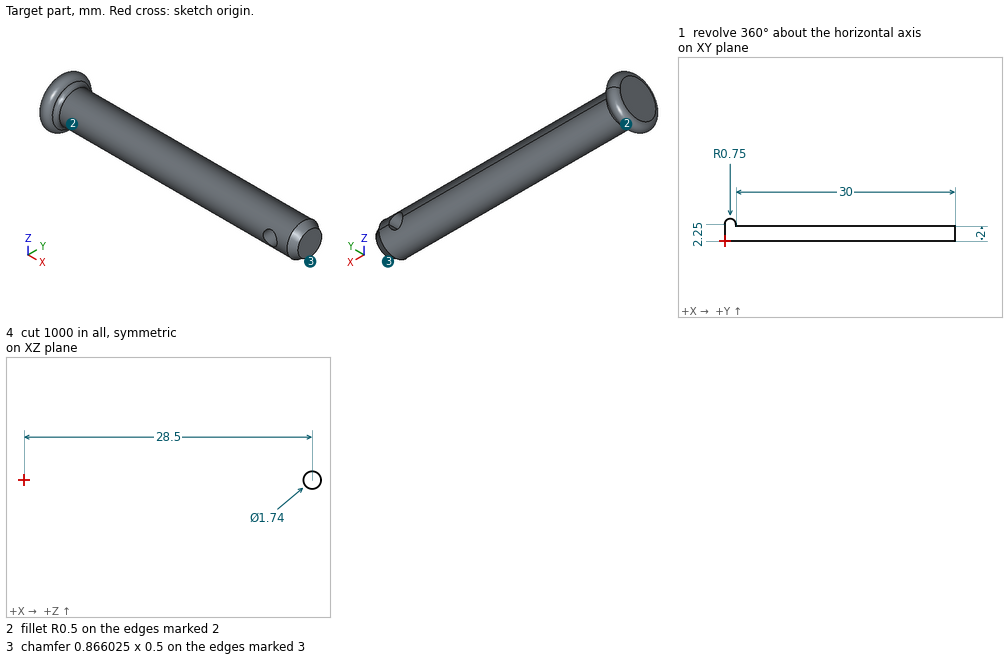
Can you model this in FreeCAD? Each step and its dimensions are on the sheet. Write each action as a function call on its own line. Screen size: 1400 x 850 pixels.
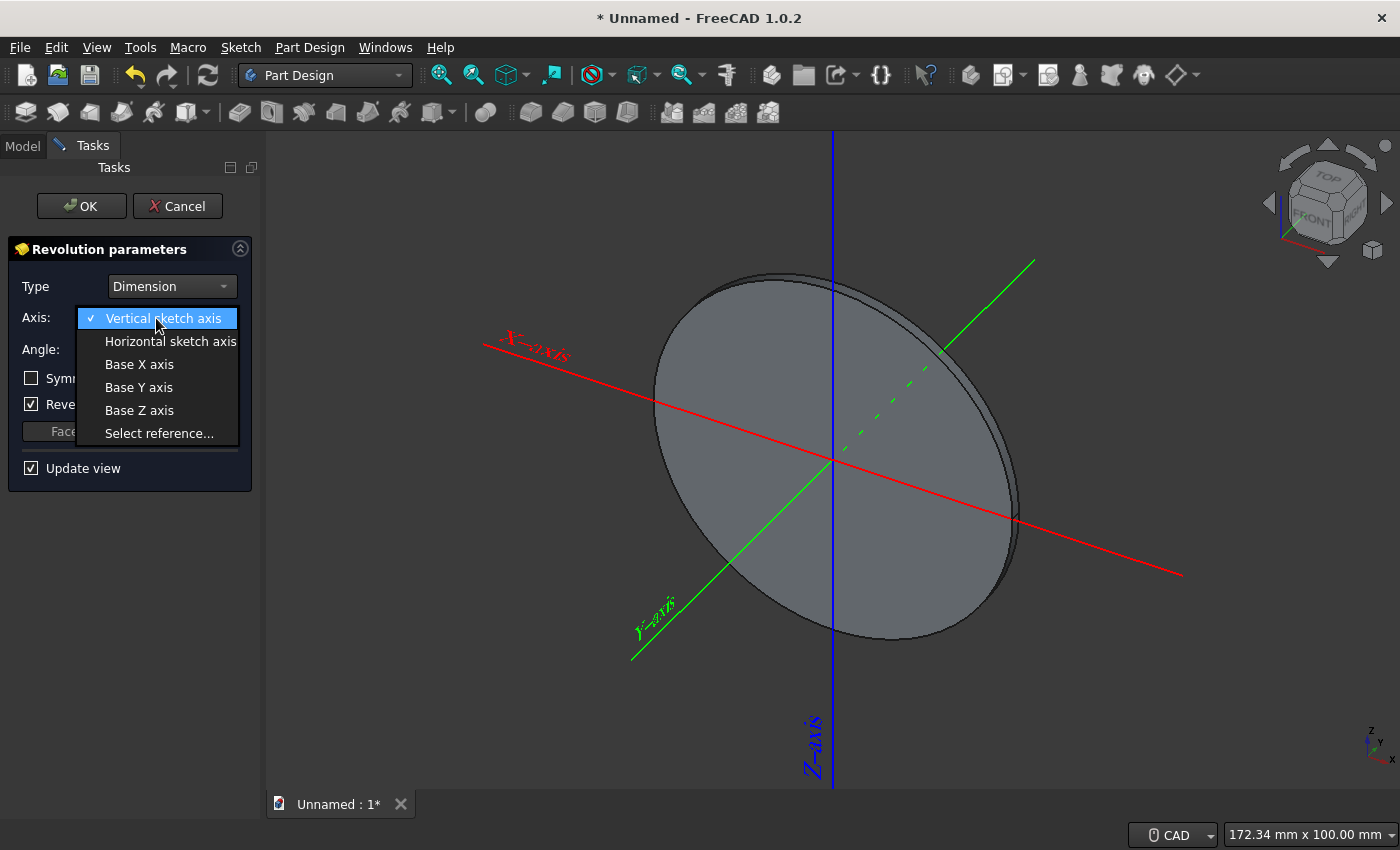
click(156, 342)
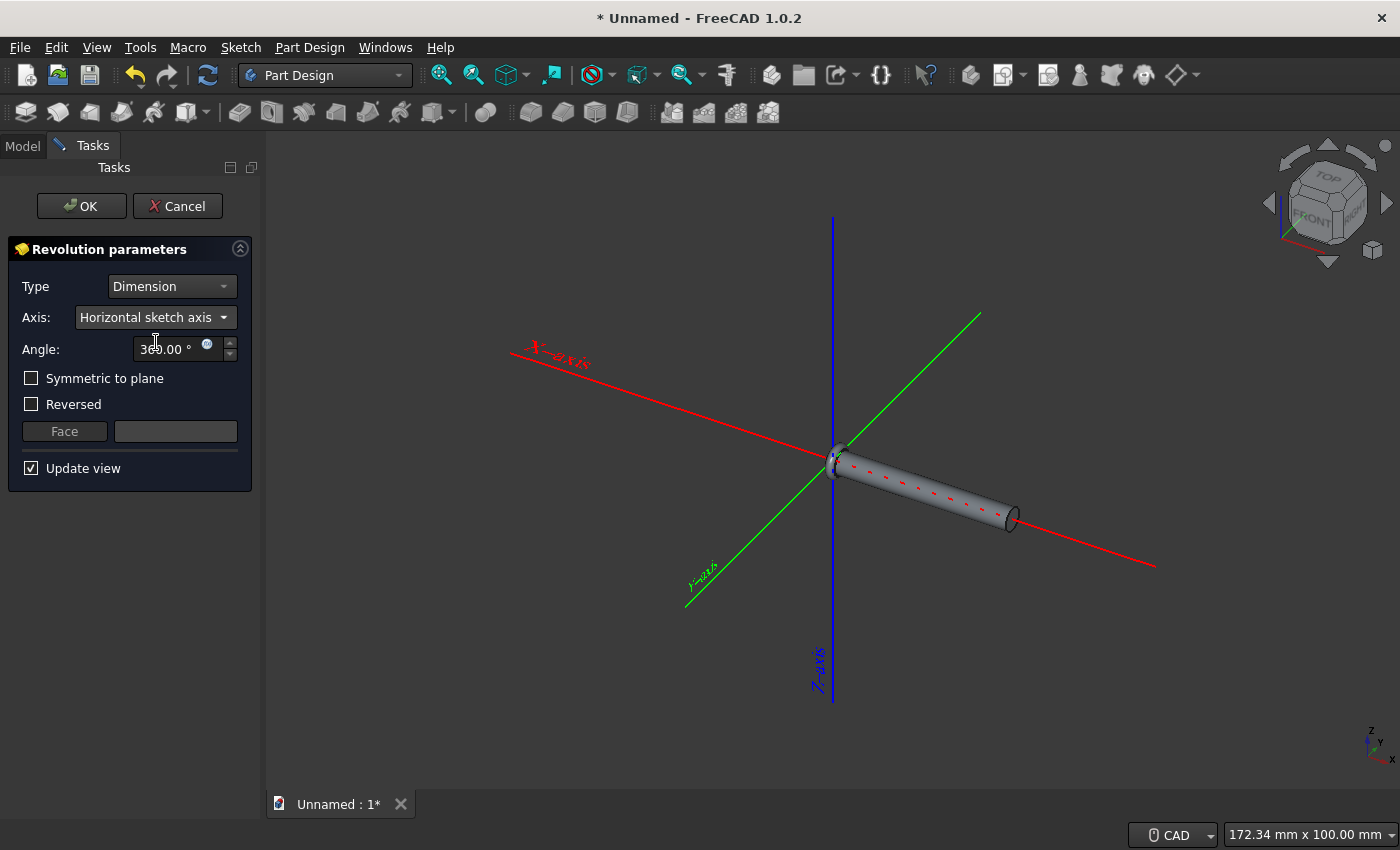
click(82, 206)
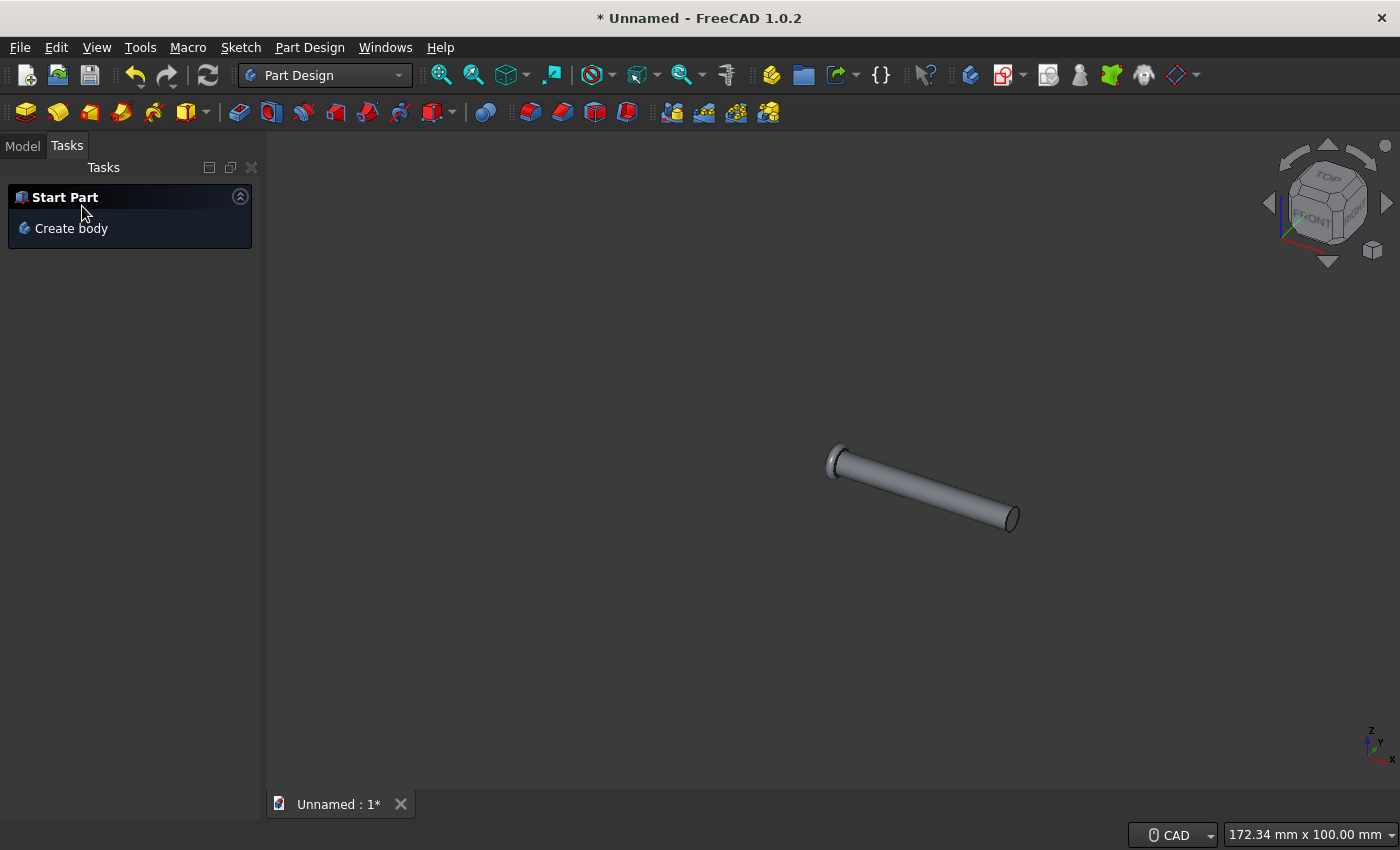
click(442, 76)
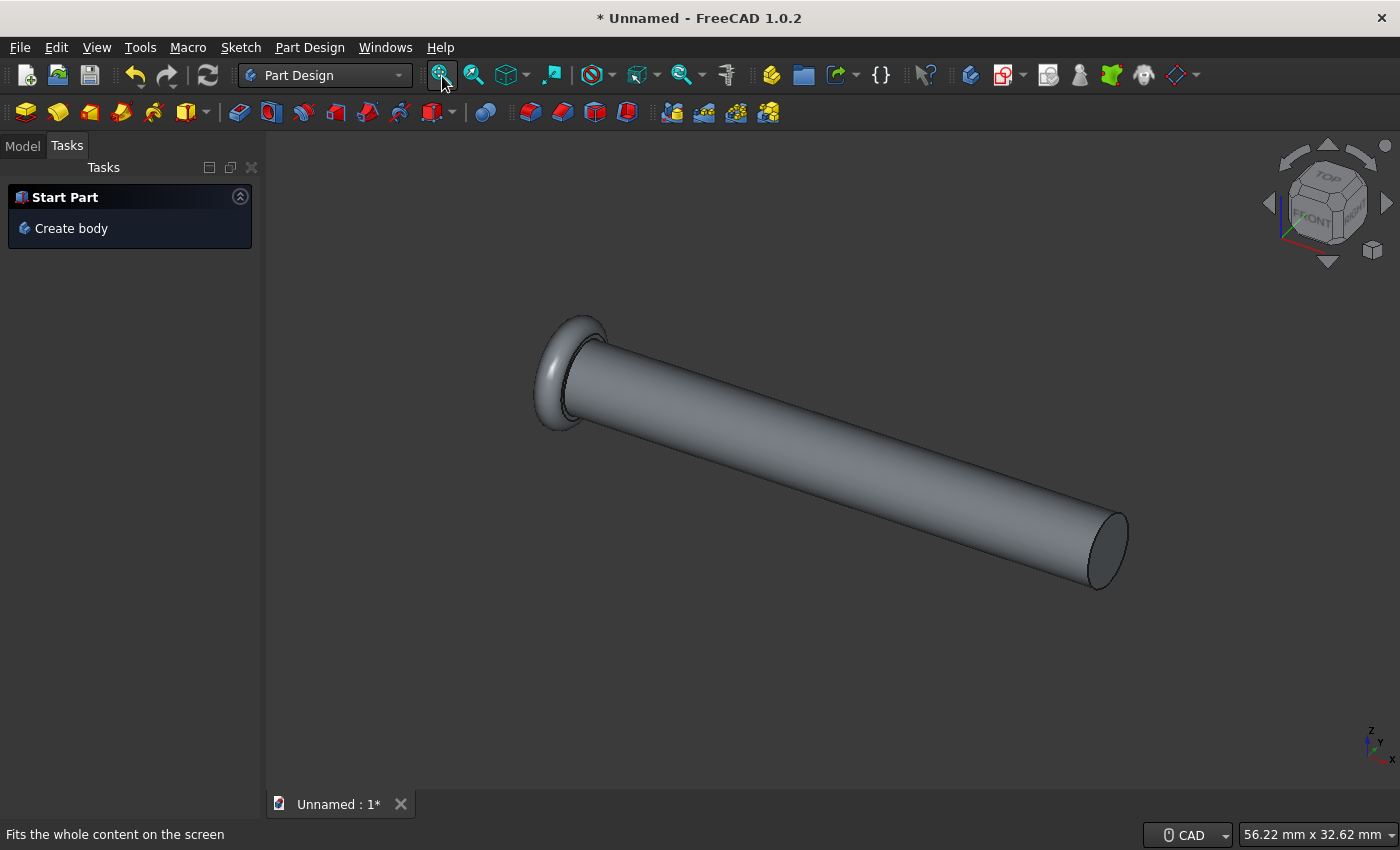
key(0)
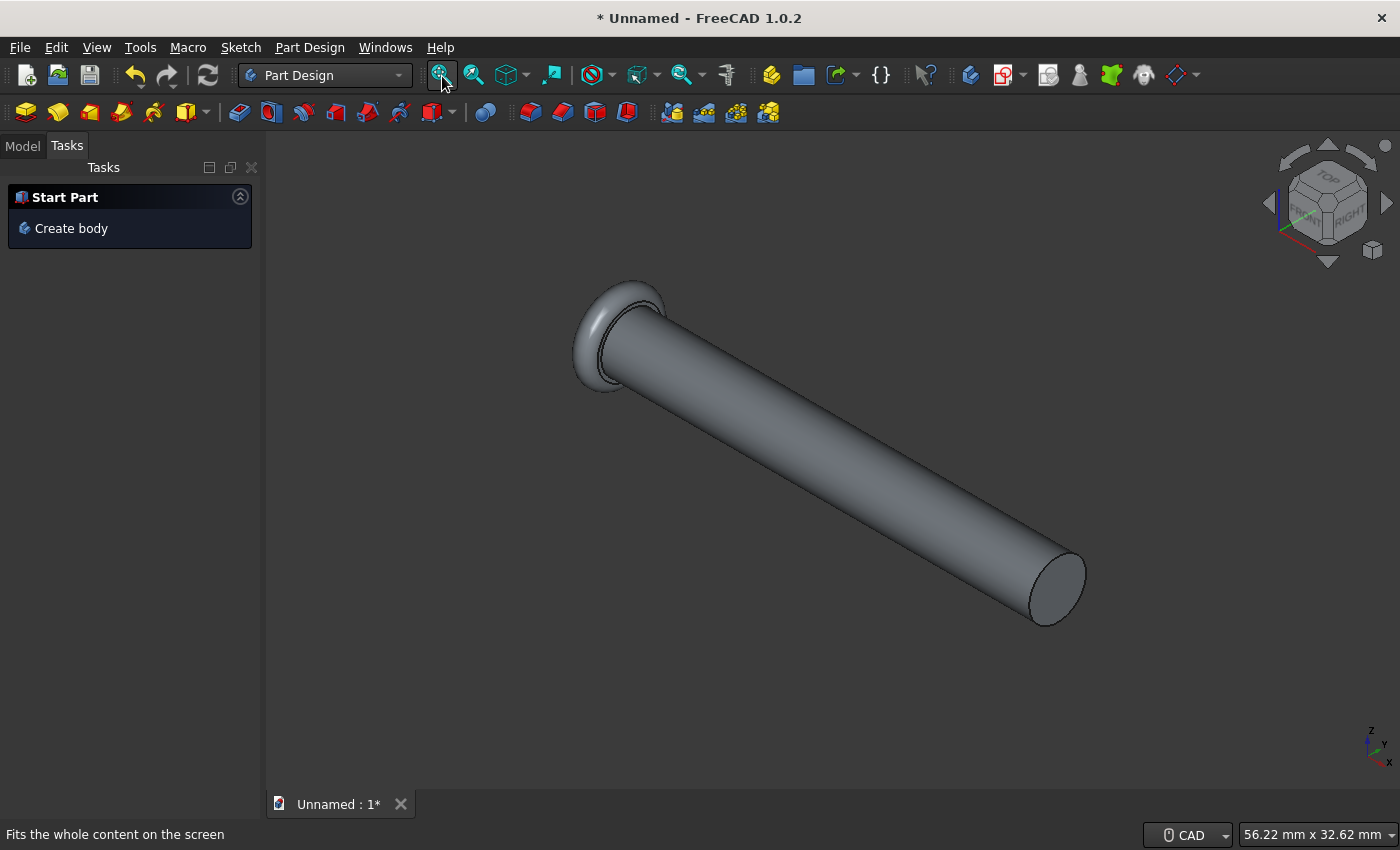
key(2)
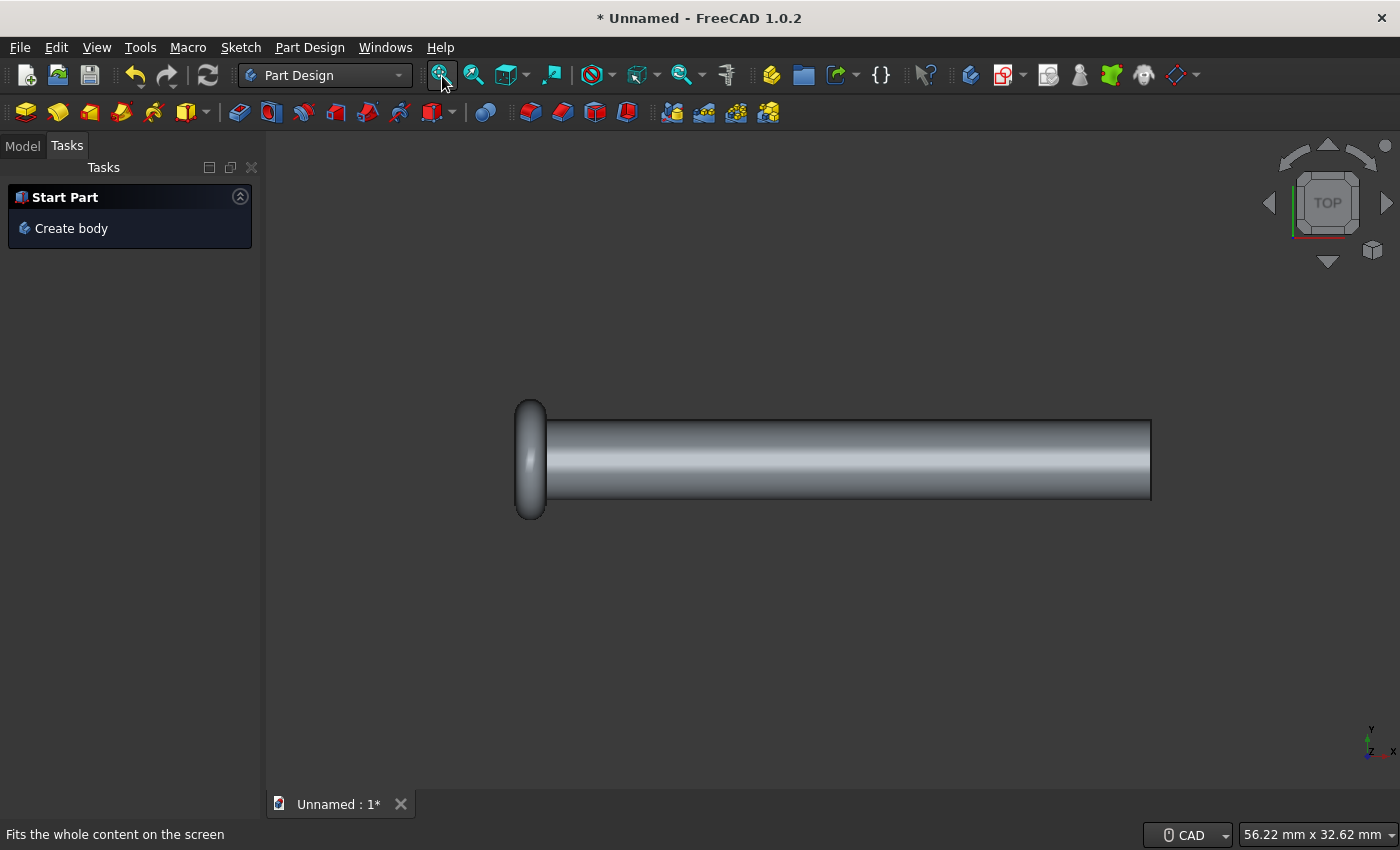
key(1)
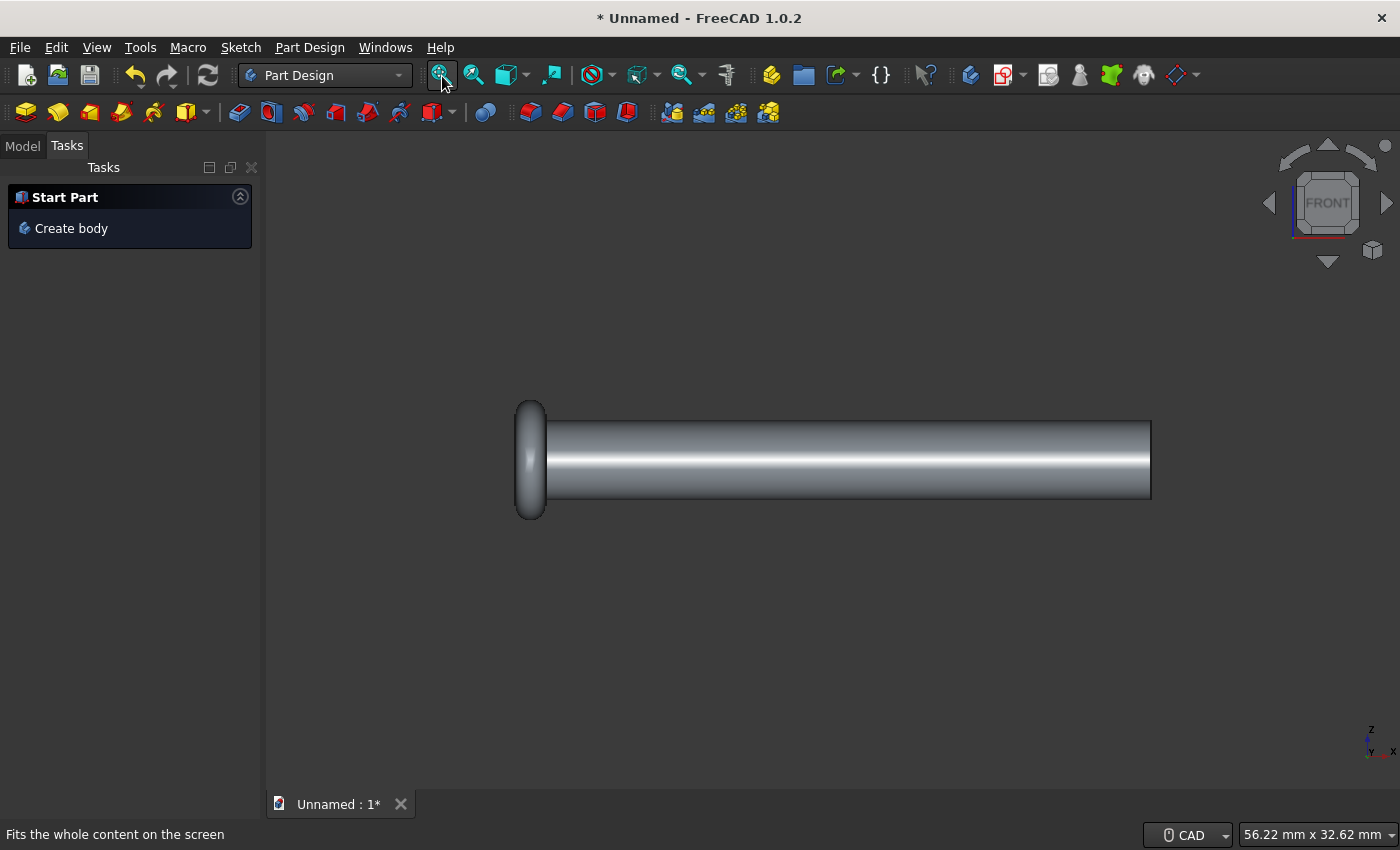
key(3)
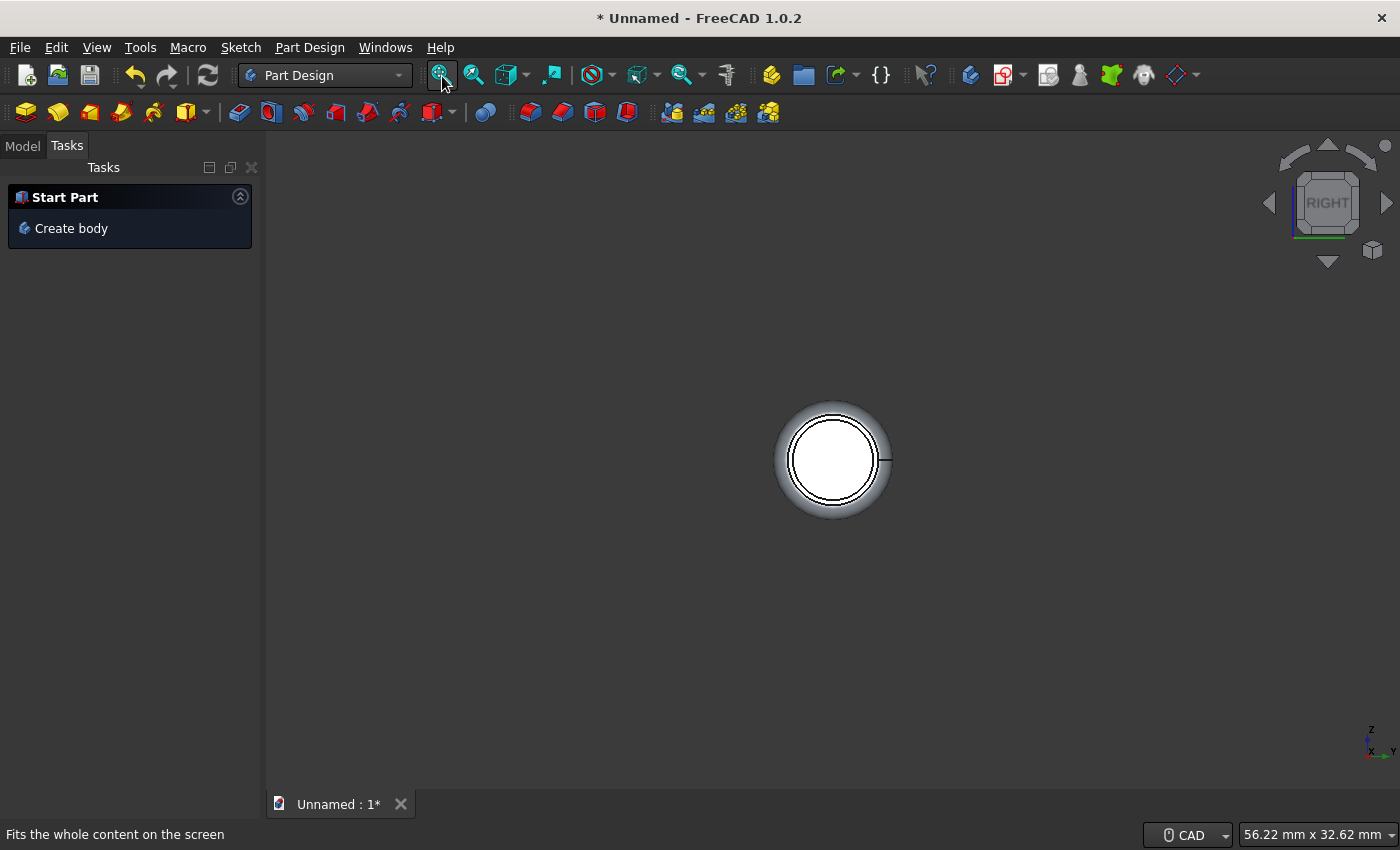
click(442, 76)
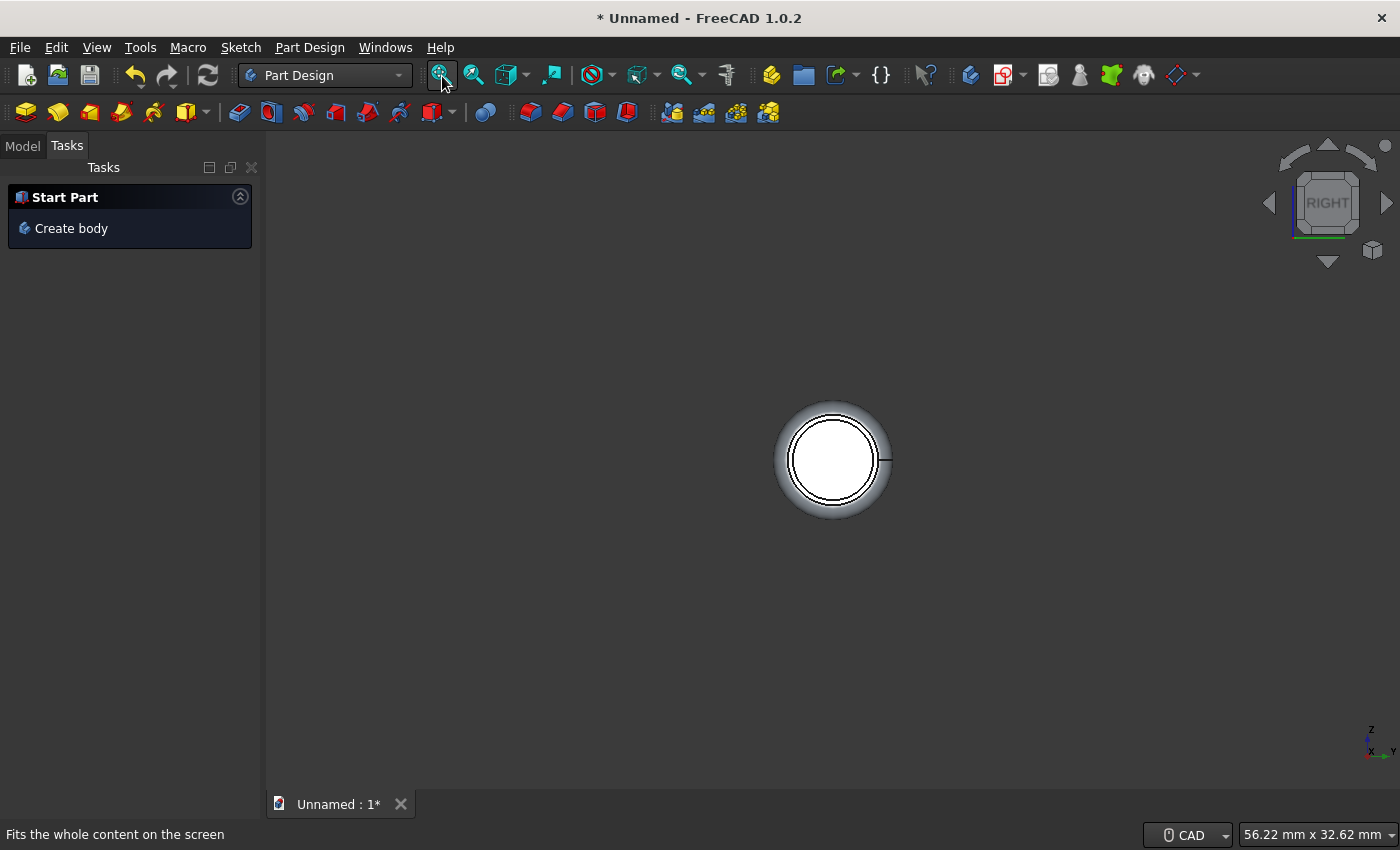
key(5)